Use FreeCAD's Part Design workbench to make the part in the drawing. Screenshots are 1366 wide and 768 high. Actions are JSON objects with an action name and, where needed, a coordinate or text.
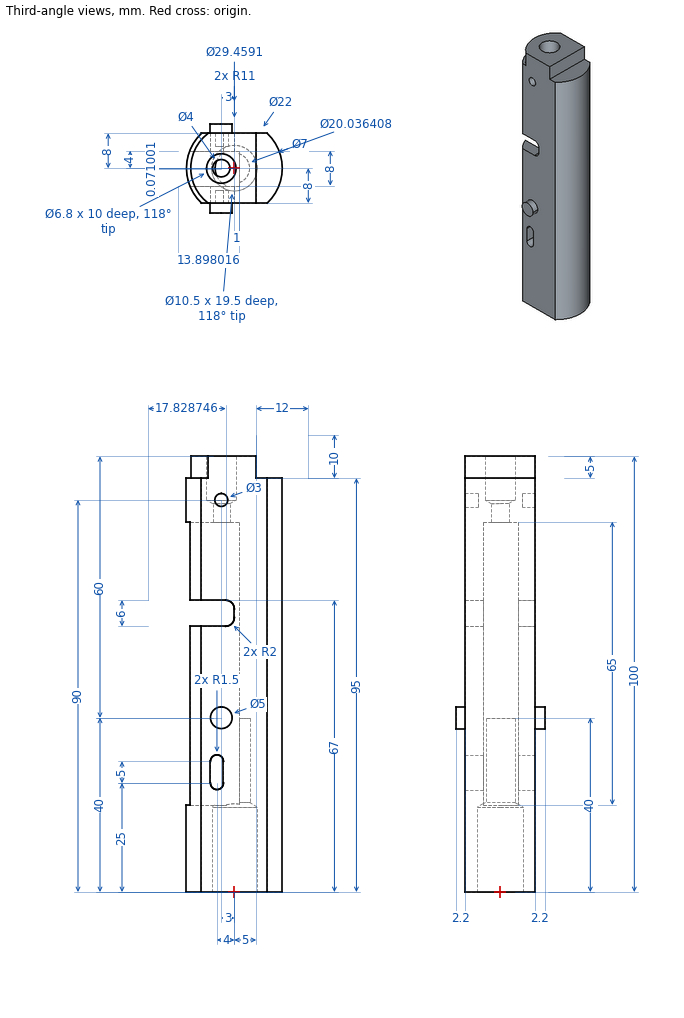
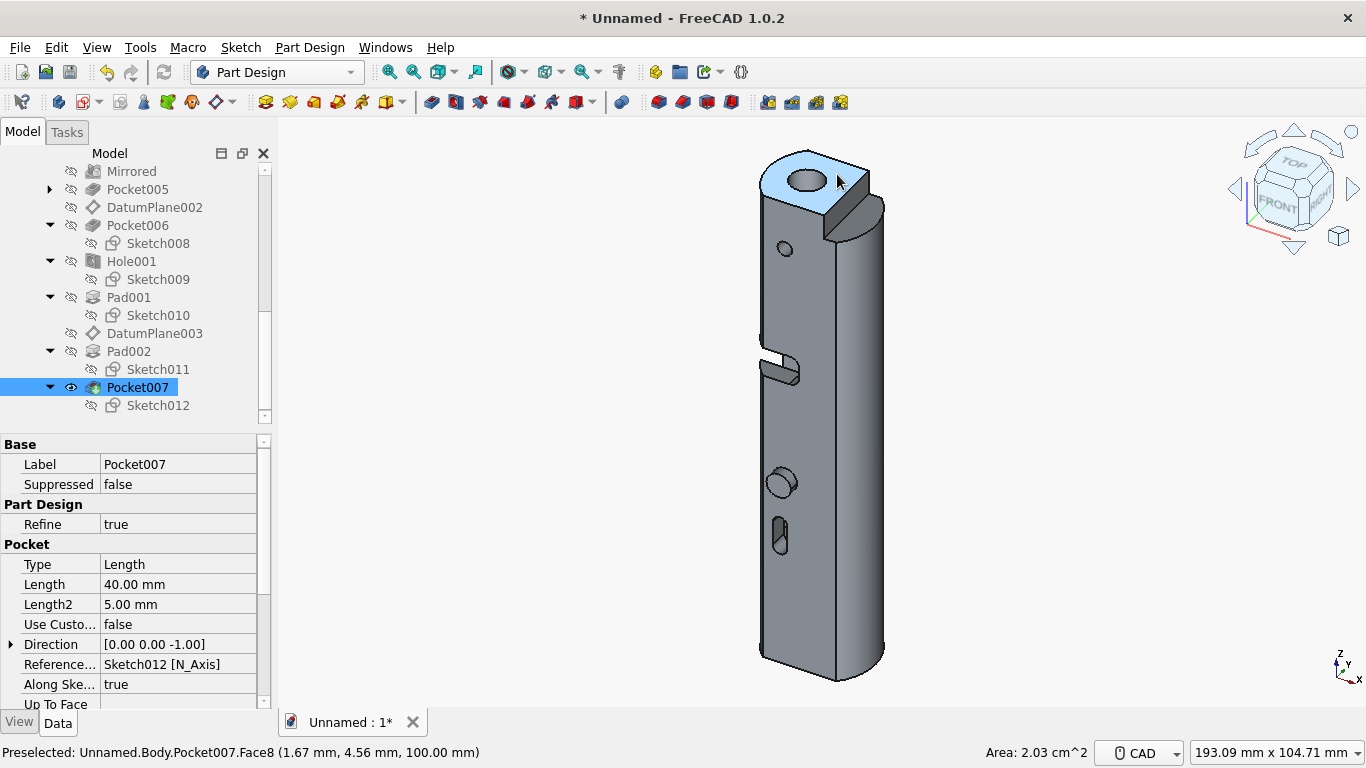
{"action": "left_click", "coordinate": [84, 102]}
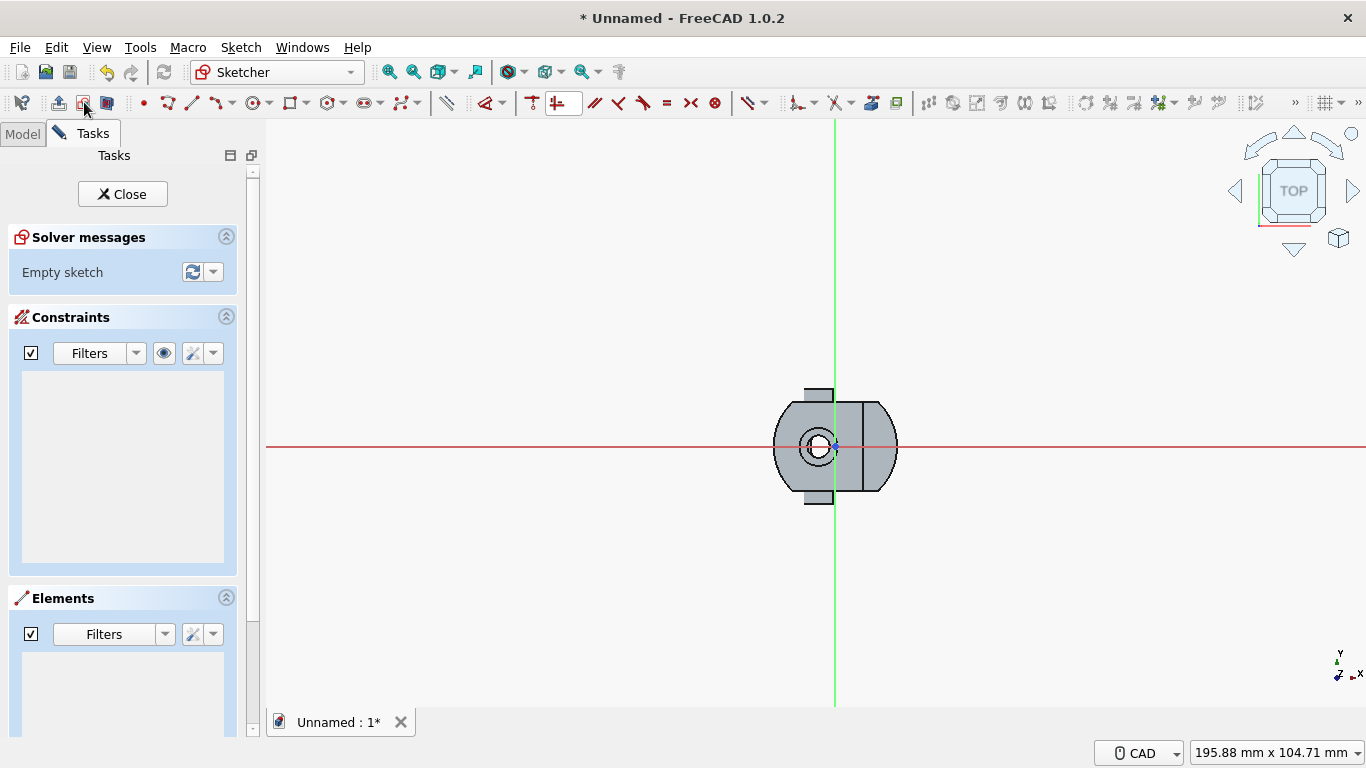
{"action": "scroll", "coordinate": [907, 474], "scroll_direction": "up", "scroll_amount": 4}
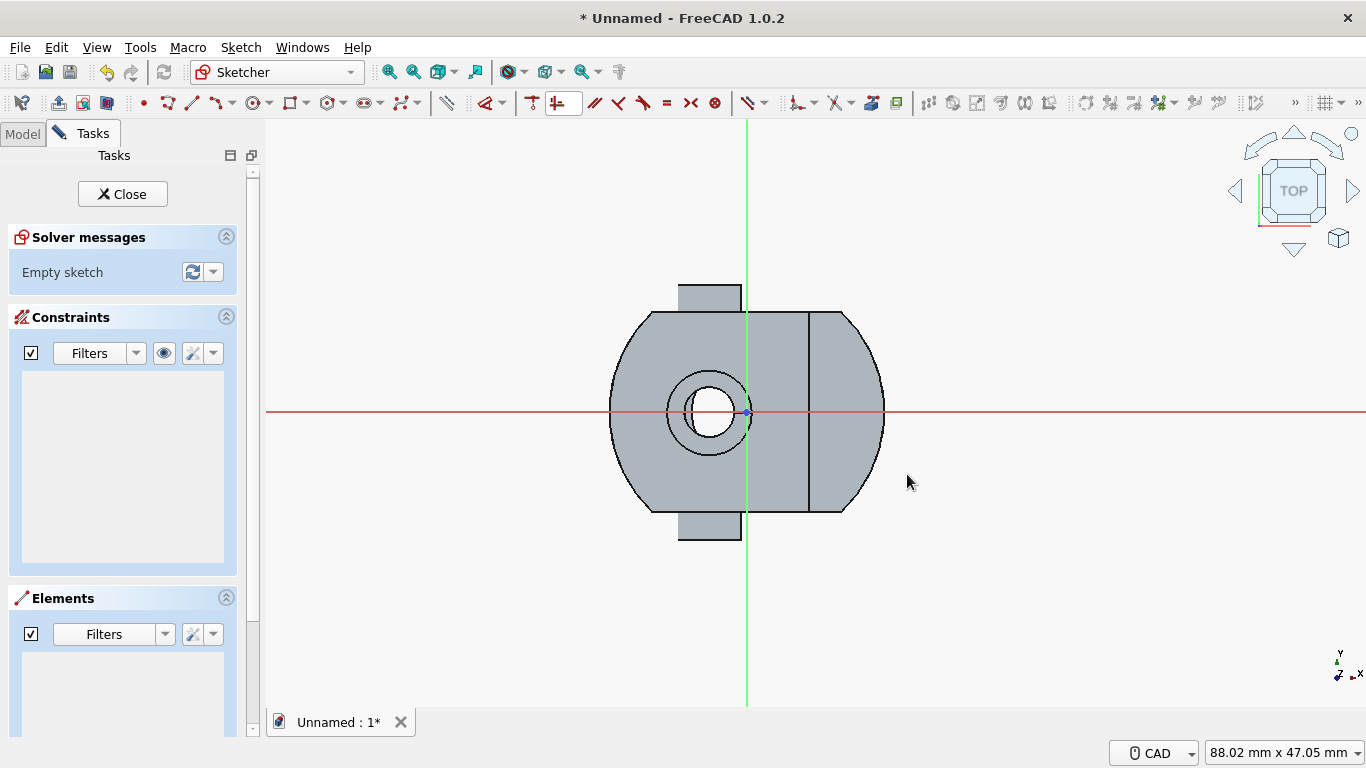
{"action": "key", "text": "g c"}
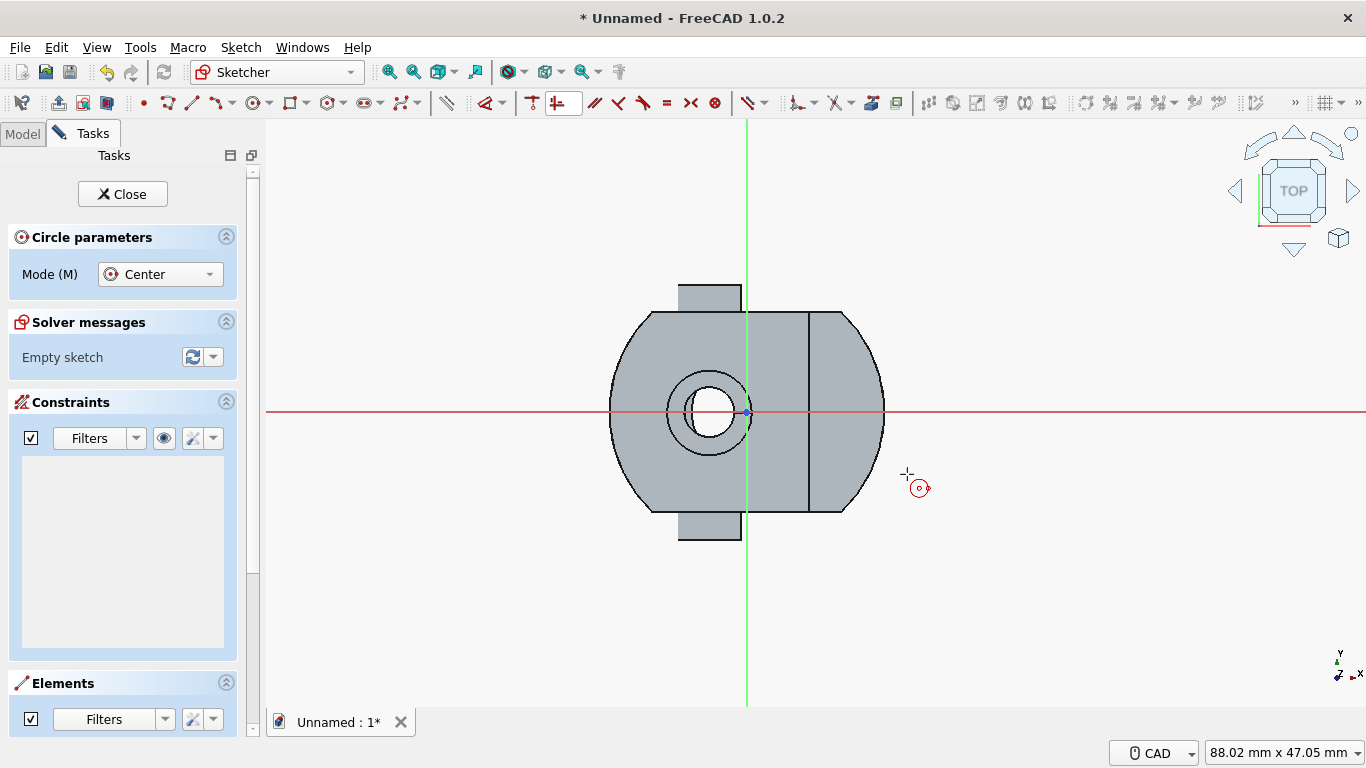
{"action": "left_click", "coordinate": [747, 412]}
{"action": "mouse_move", "coordinate": [877, 282]}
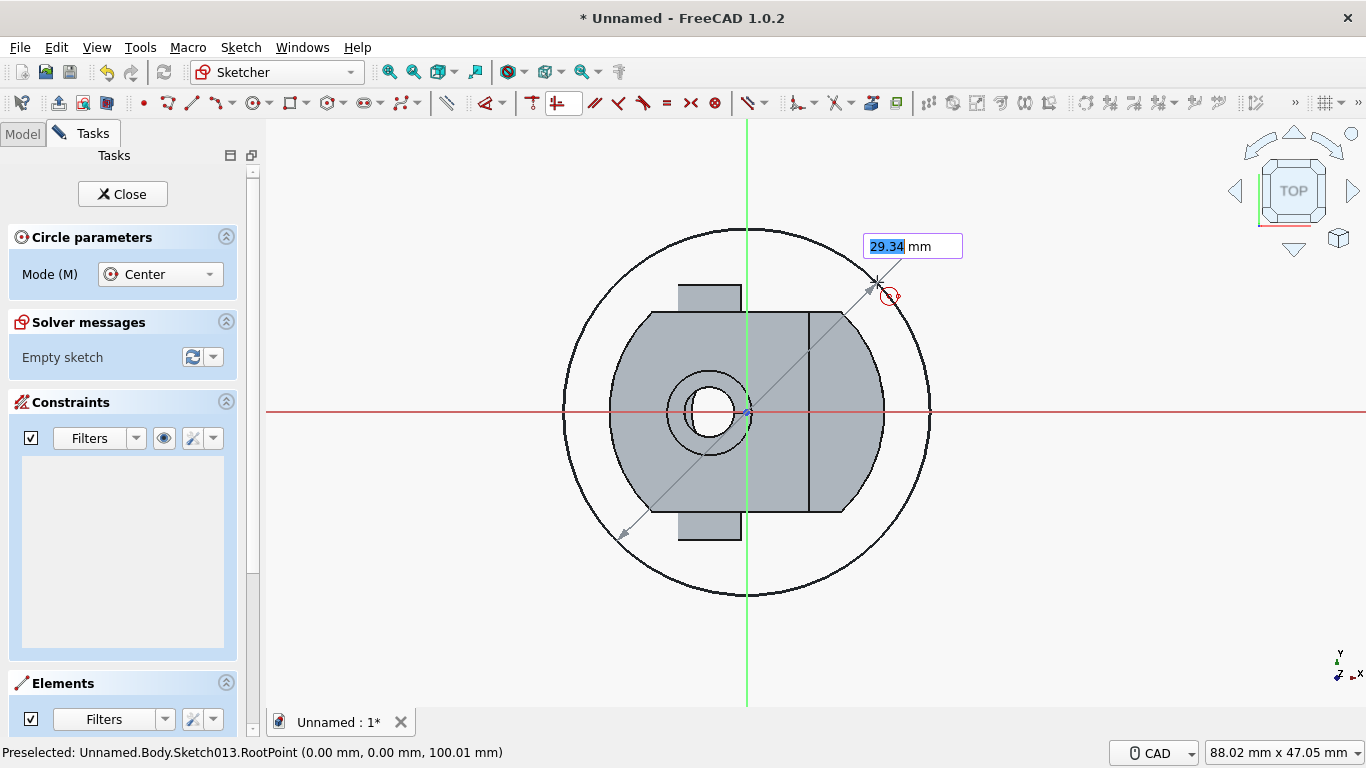
{"action": "type", "text": "29.4591"}
{"action": "key", "text": "Return"}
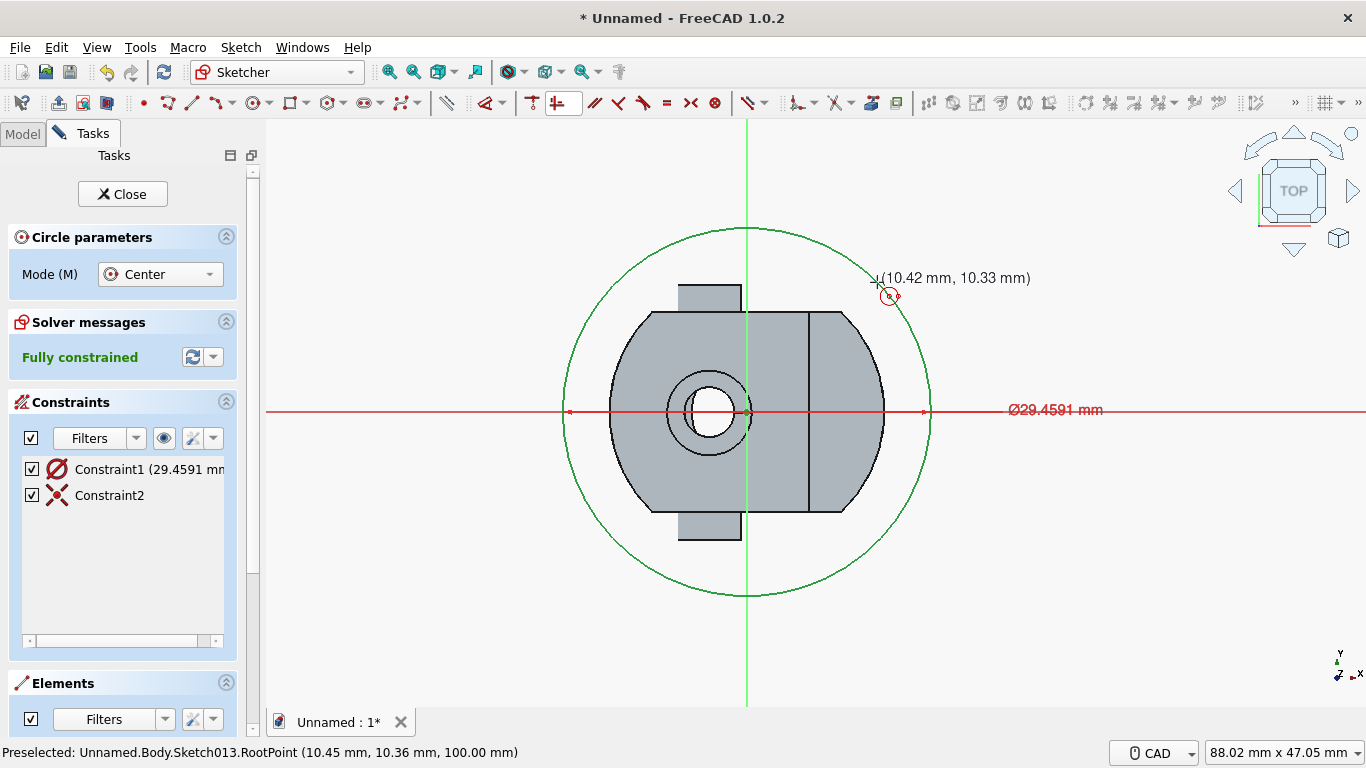
{"action": "left_click", "coordinate": [747, 412]}
{"action": "mouse_move", "coordinate": [835, 324]}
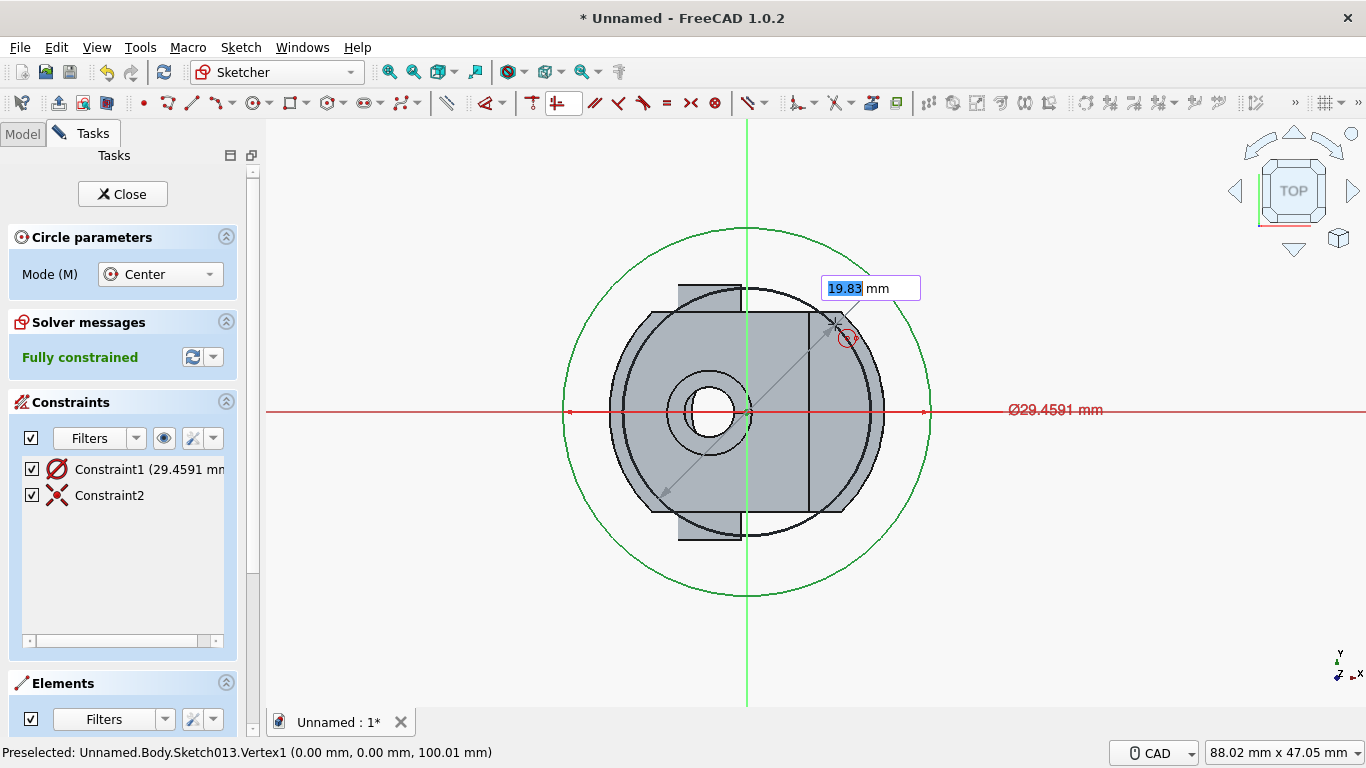
{"action": "type", "text": "20.036408"}
{"action": "key", "text": "Return"}
{"action": "key", "text": "Escape"}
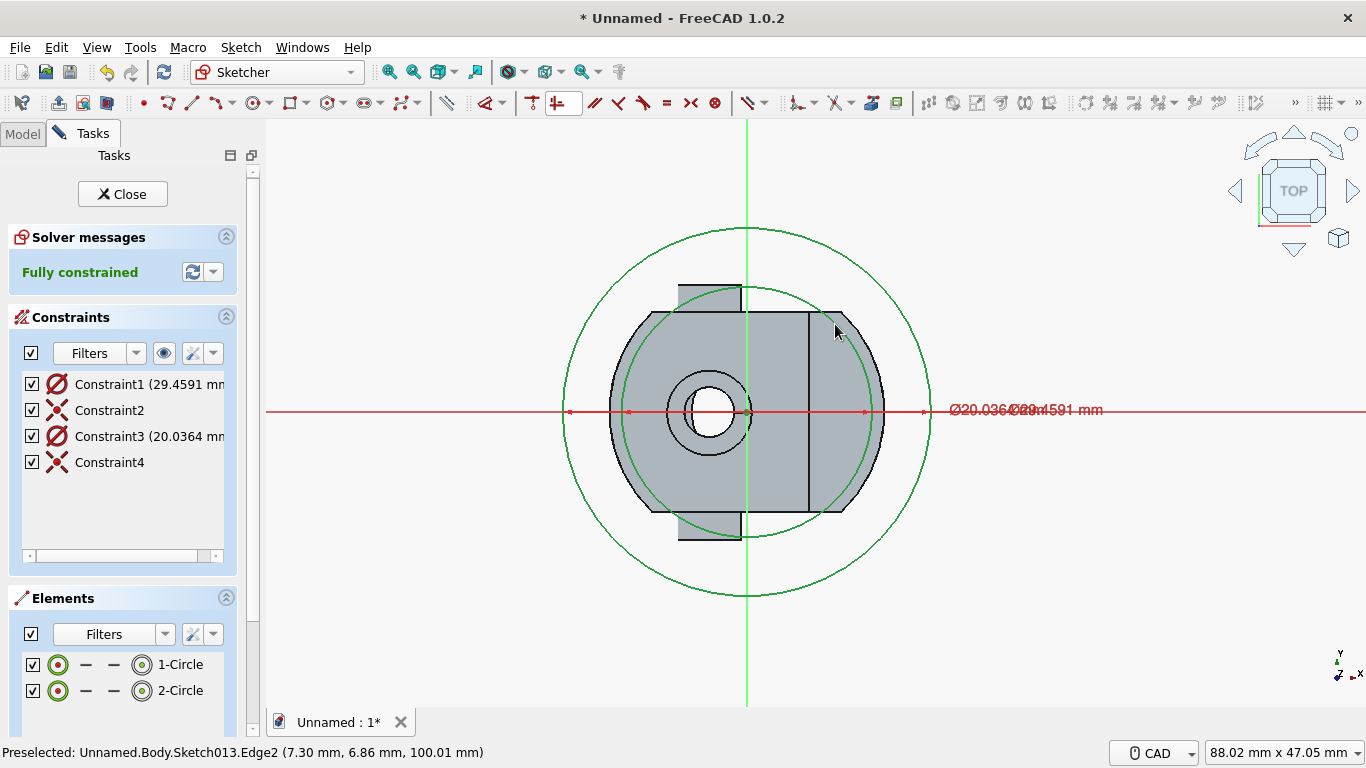
{"action": "left_click", "coordinate": [123, 194]}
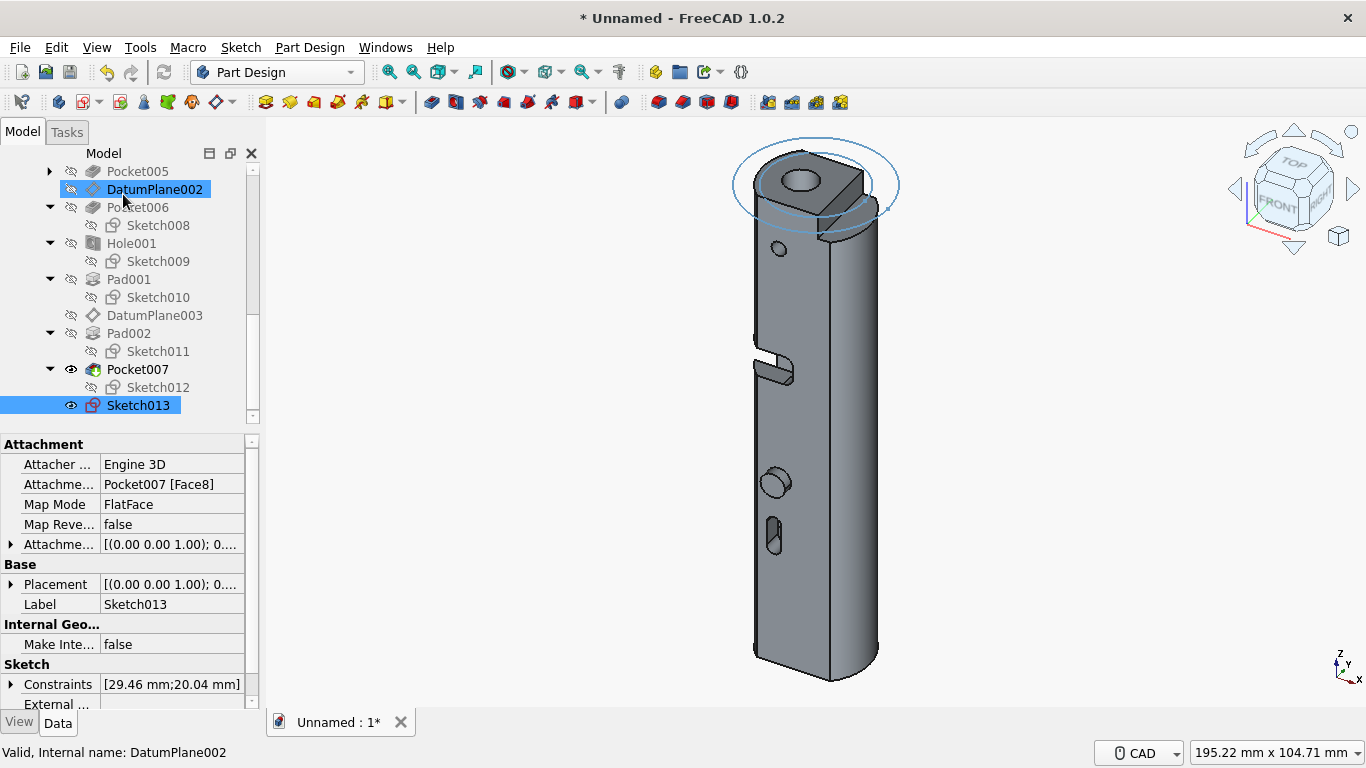
{"action": "left_click", "coordinate": [432, 102]}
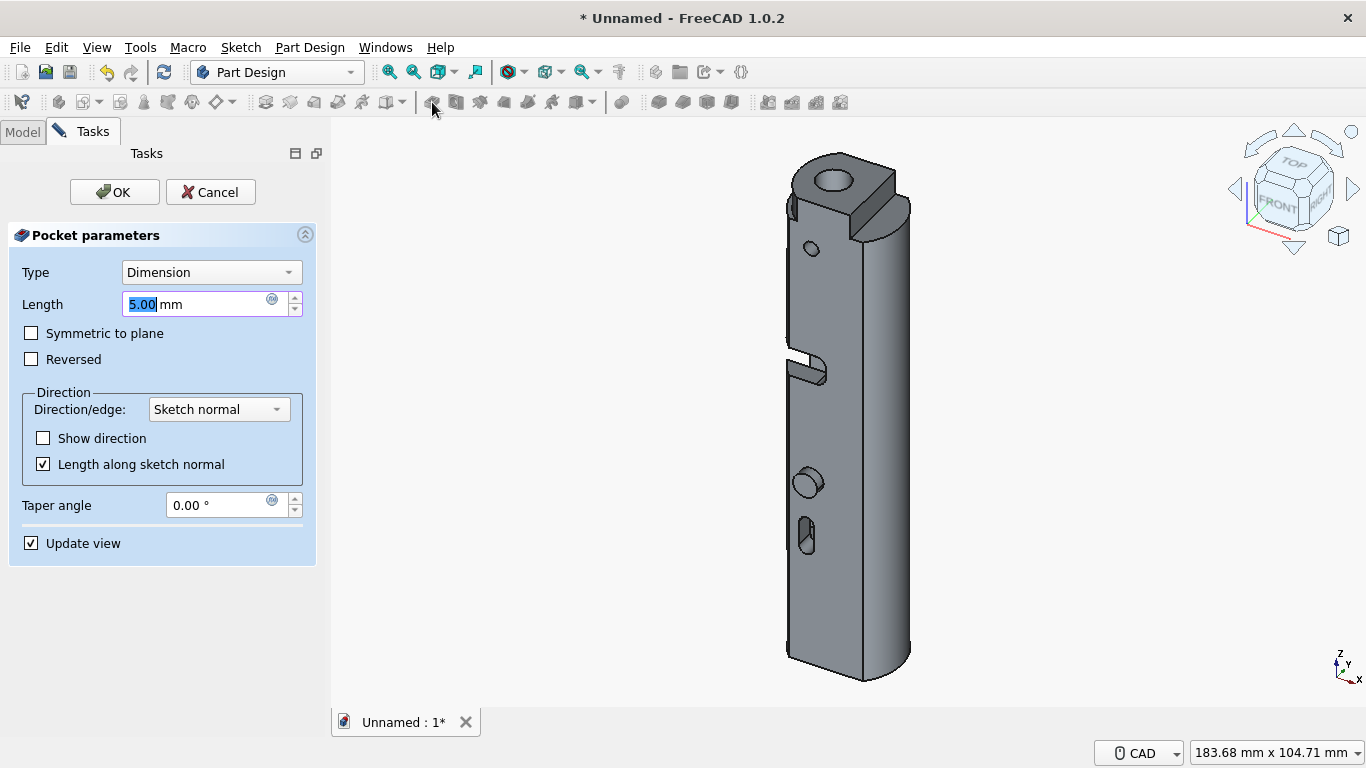
{"action": "type", "text": "5"}
{"action": "key", "text": "Tab"}